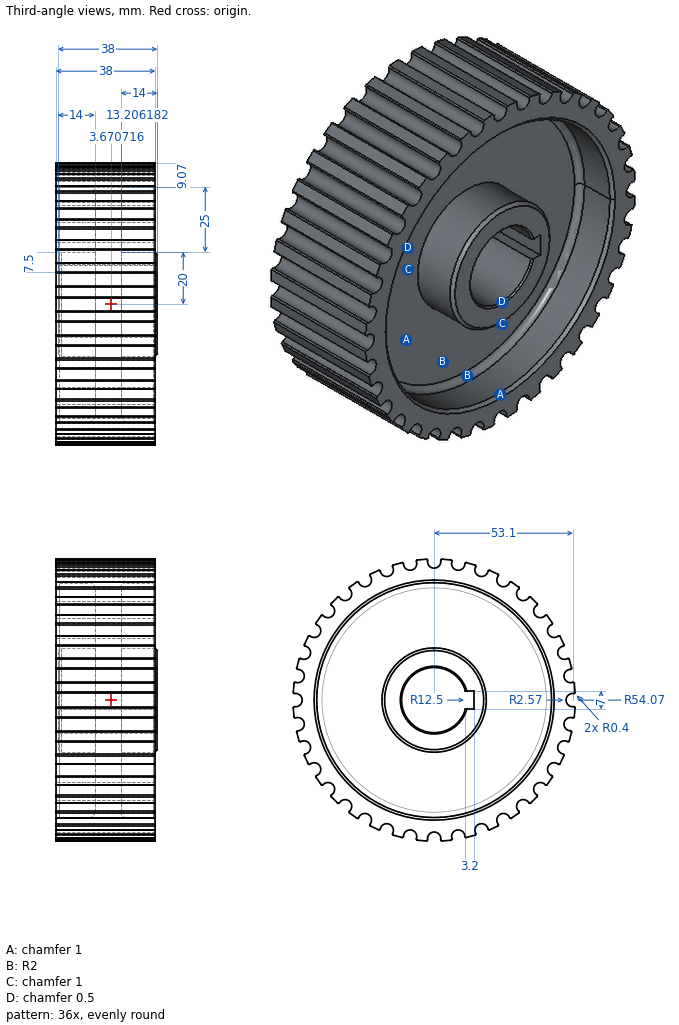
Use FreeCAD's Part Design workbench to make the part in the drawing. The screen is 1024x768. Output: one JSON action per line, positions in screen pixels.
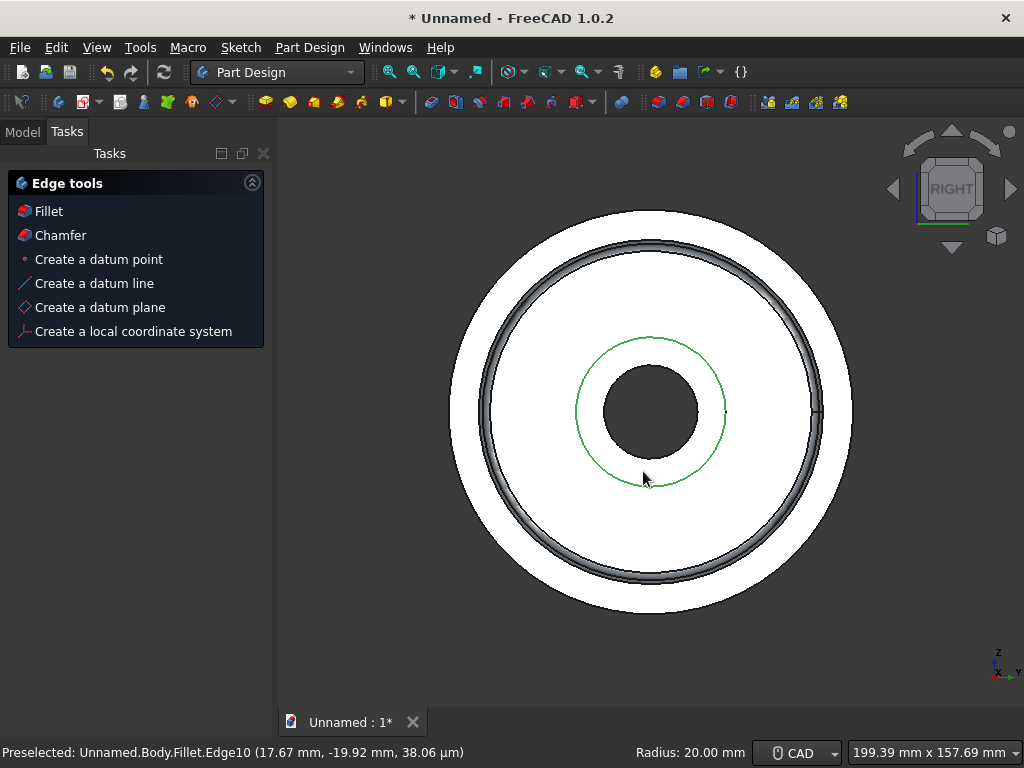
{"action": "key", "text": "5"}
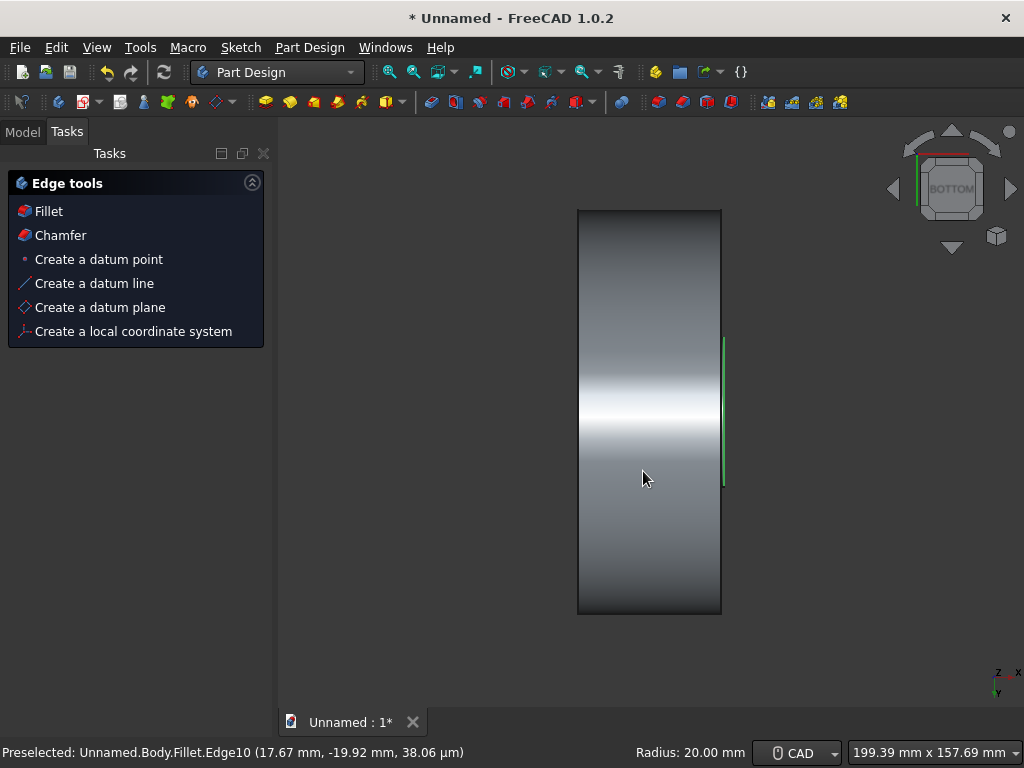
{"action": "key", "text": "4"}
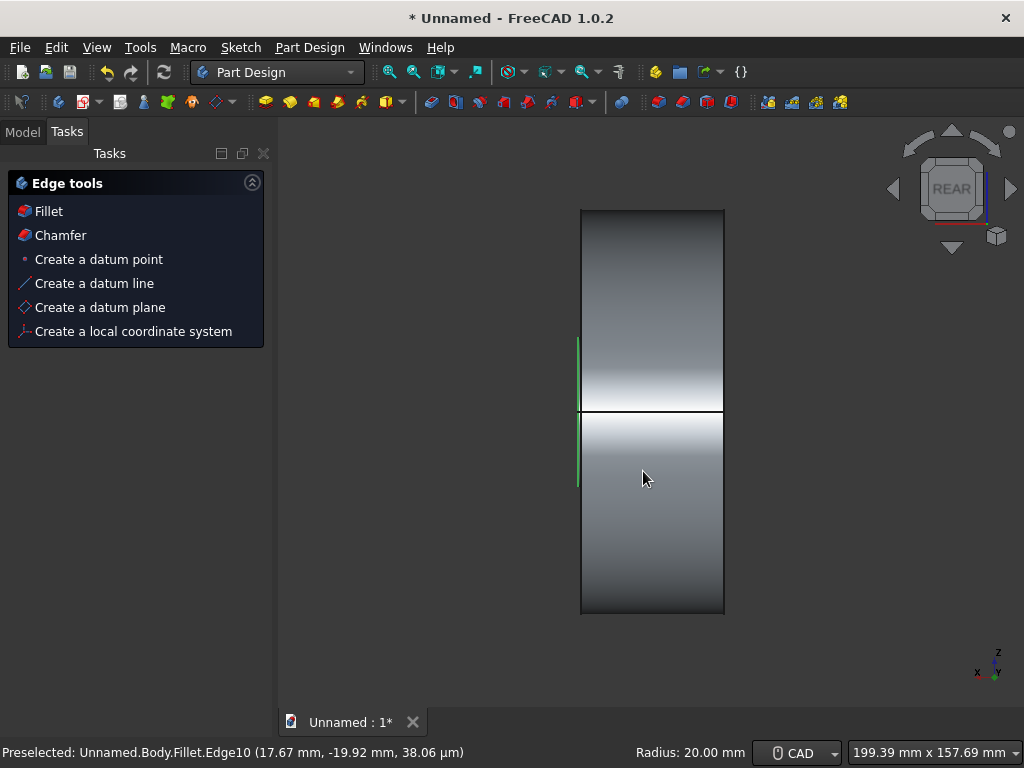
{"action": "key", "text": "6"}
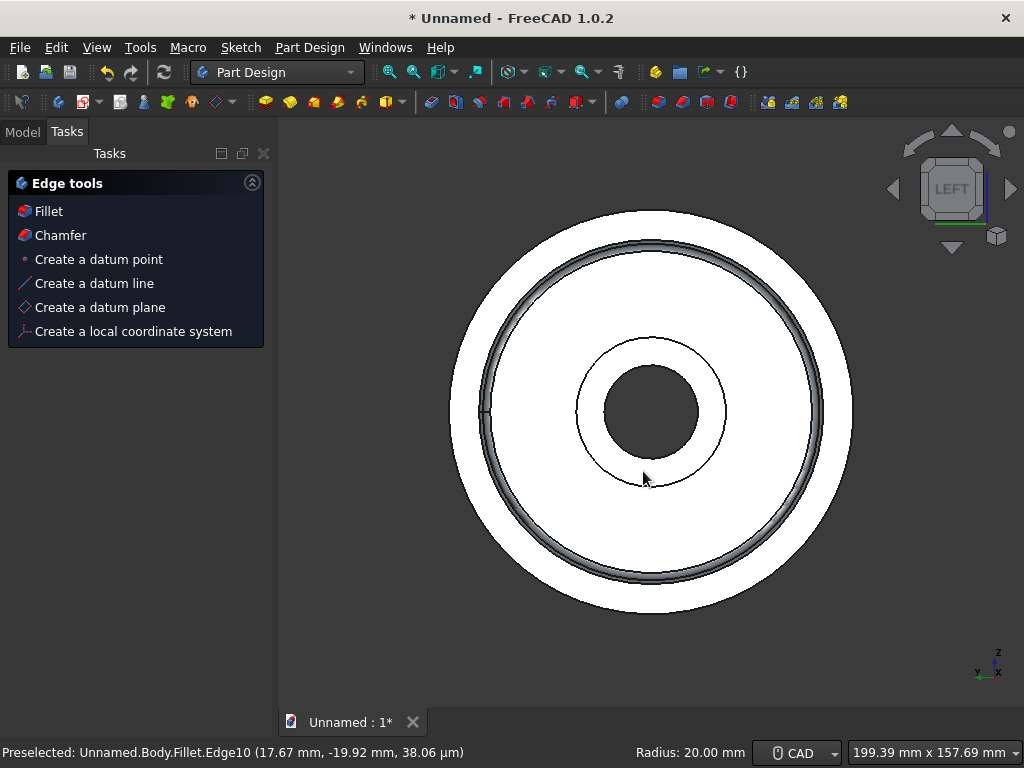
{"action": "left_click", "coordinate": [726, 411], "text": "ctrl"}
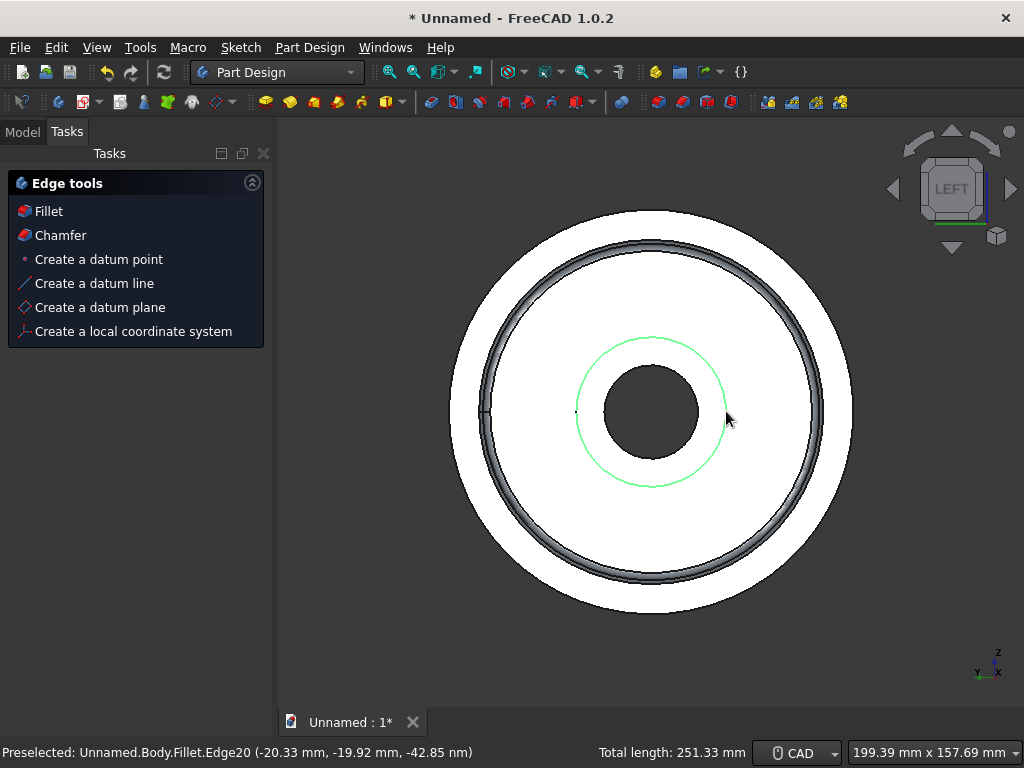
{"action": "left_click", "coordinate": [684, 102]}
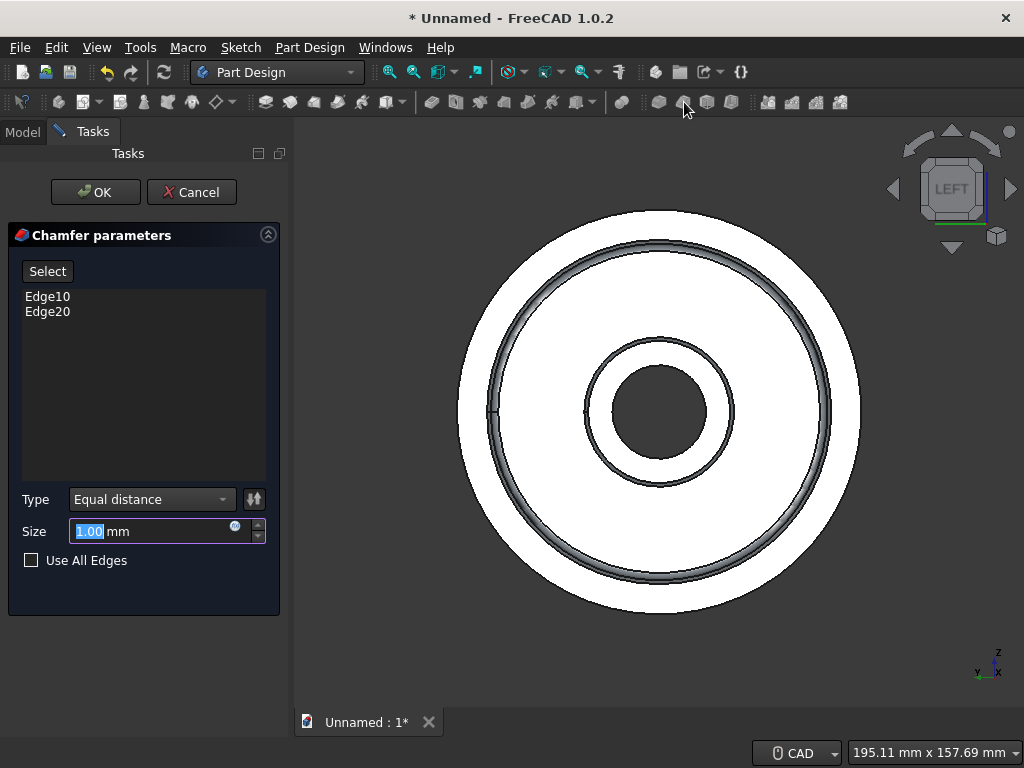
{"action": "type", "text": "1"}
{"action": "key", "text": "Tab"}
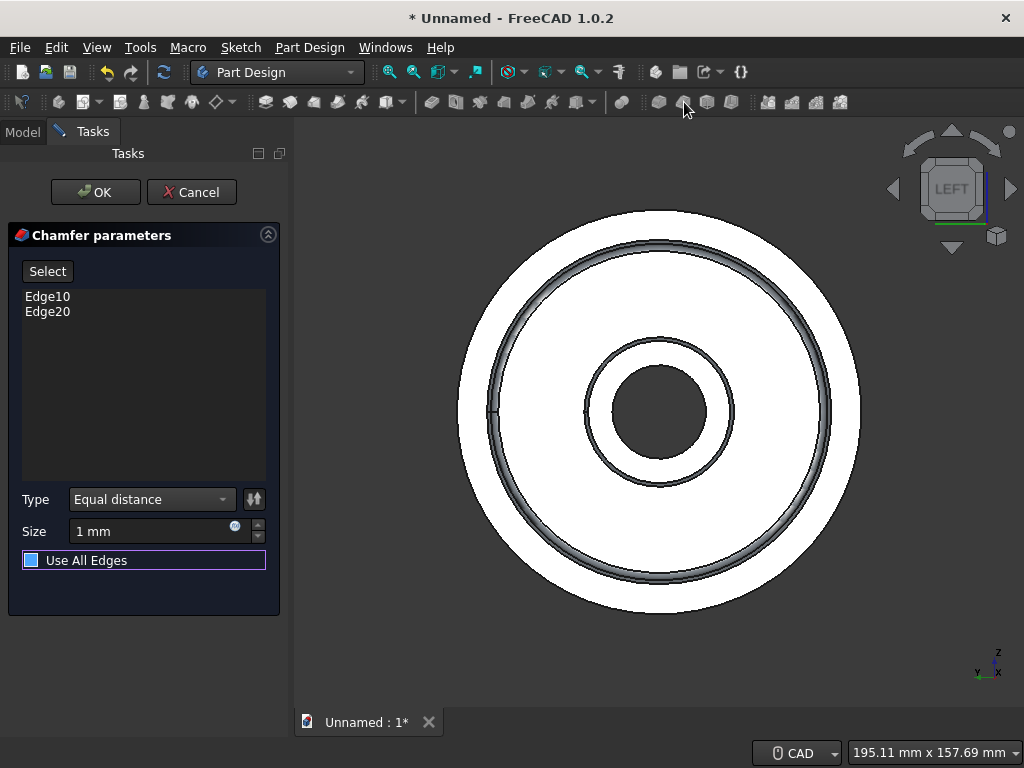
{"action": "left_click", "coordinate": [96, 192]}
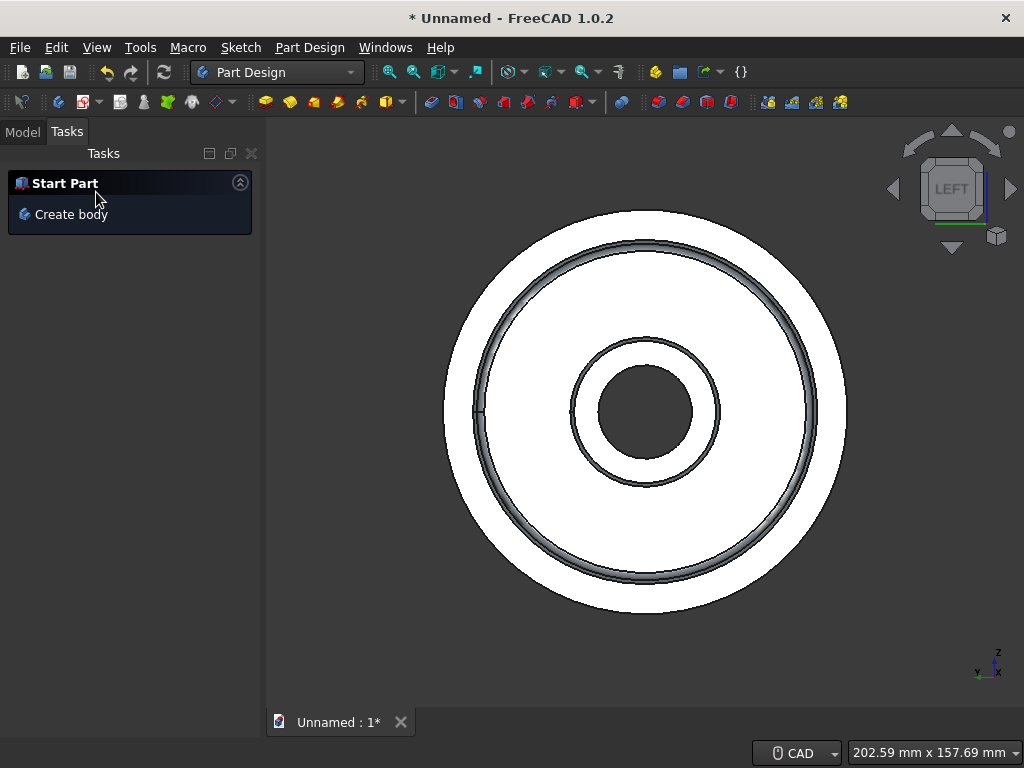
{"action": "left_click", "coordinate": [692, 411]}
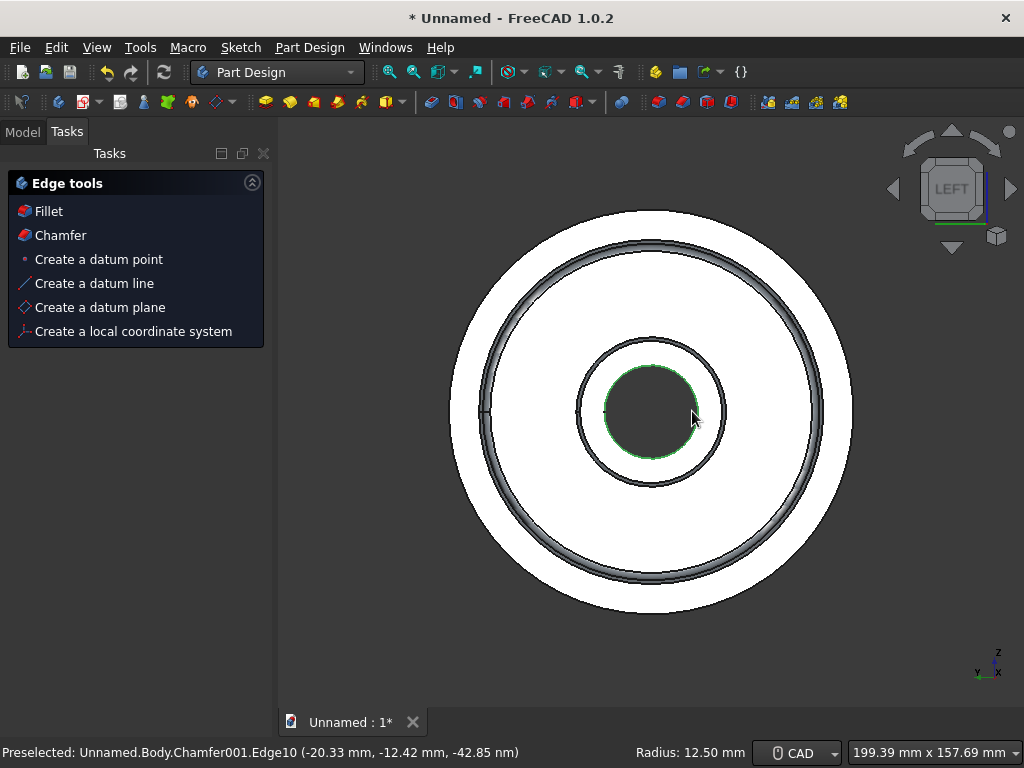
{"action": "key", "text": "0"}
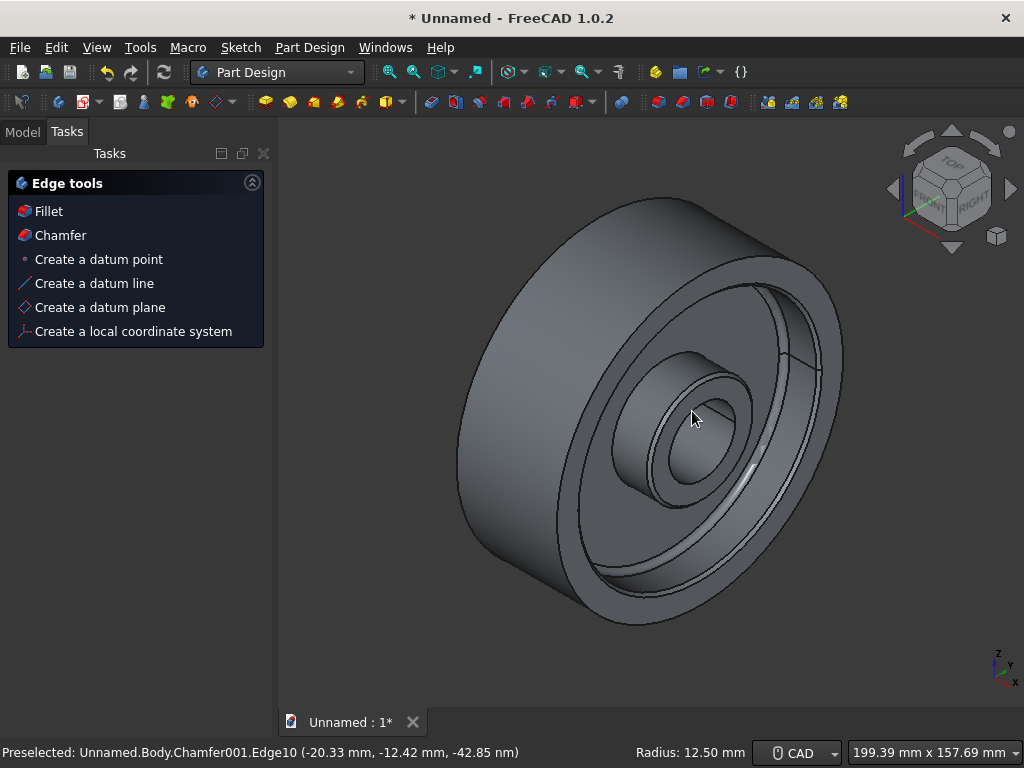
{"action": "left_click", "coordinate": [692, 483], "text": "ctrl"}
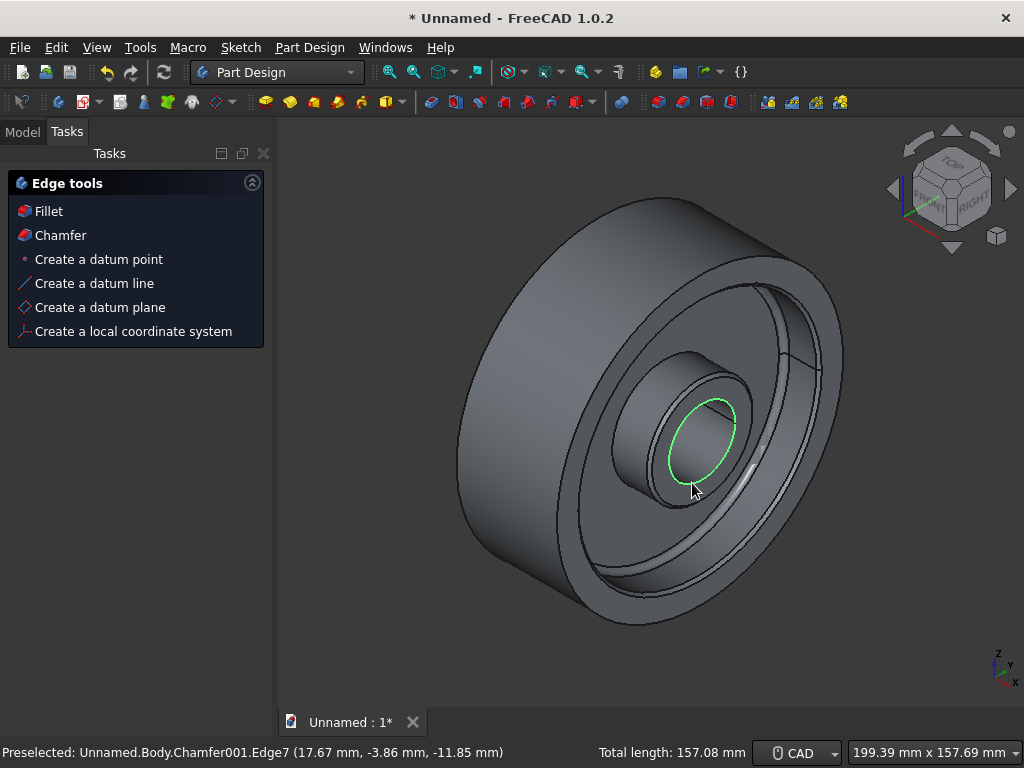
{"action": "left_click", "coordinate": [684, 102]}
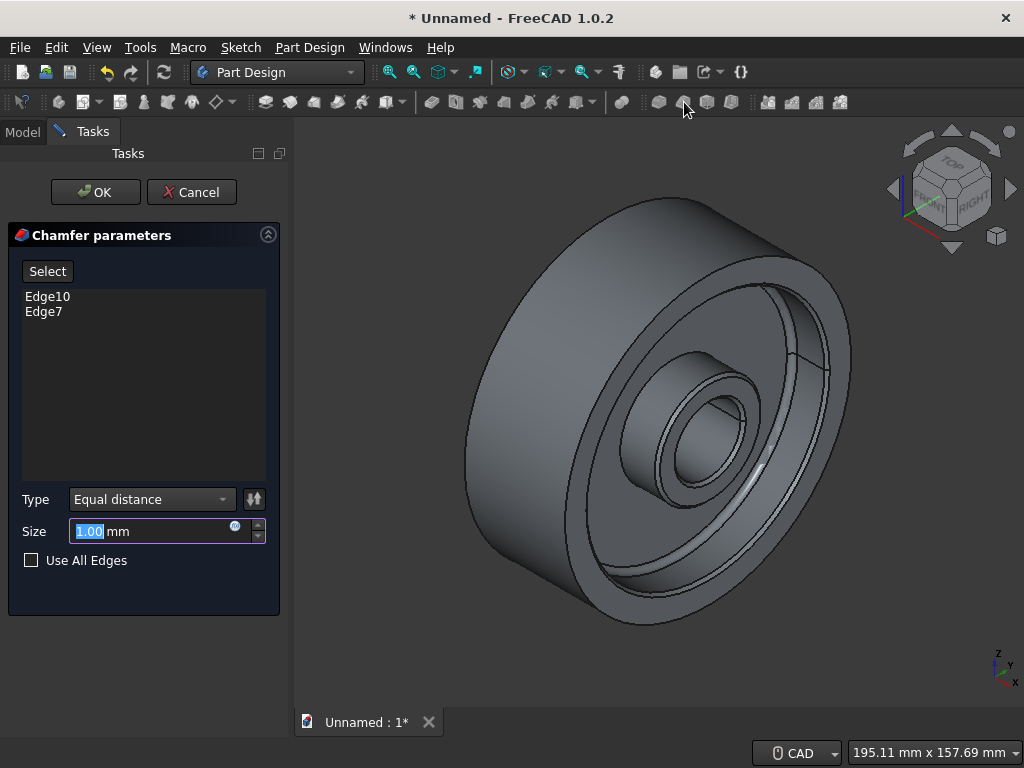
{"action": "type", "text": "0.5"}
{"action": "key", "text": "Tab"}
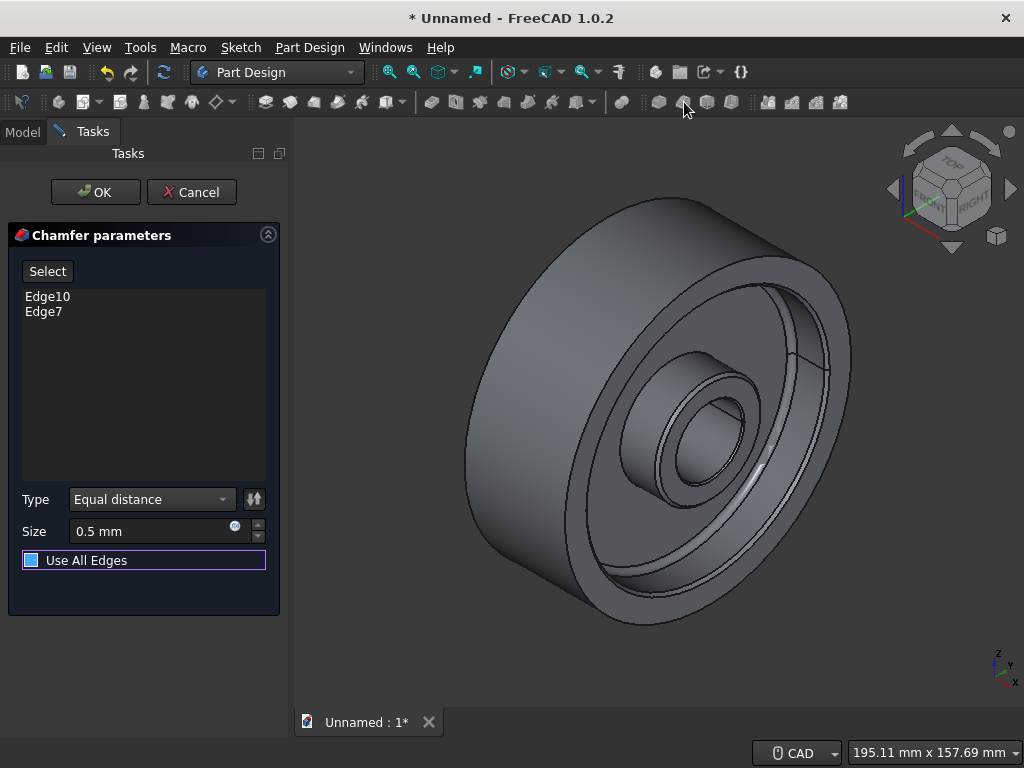
{"action": "left_click", "coordinate": [96, 192]}